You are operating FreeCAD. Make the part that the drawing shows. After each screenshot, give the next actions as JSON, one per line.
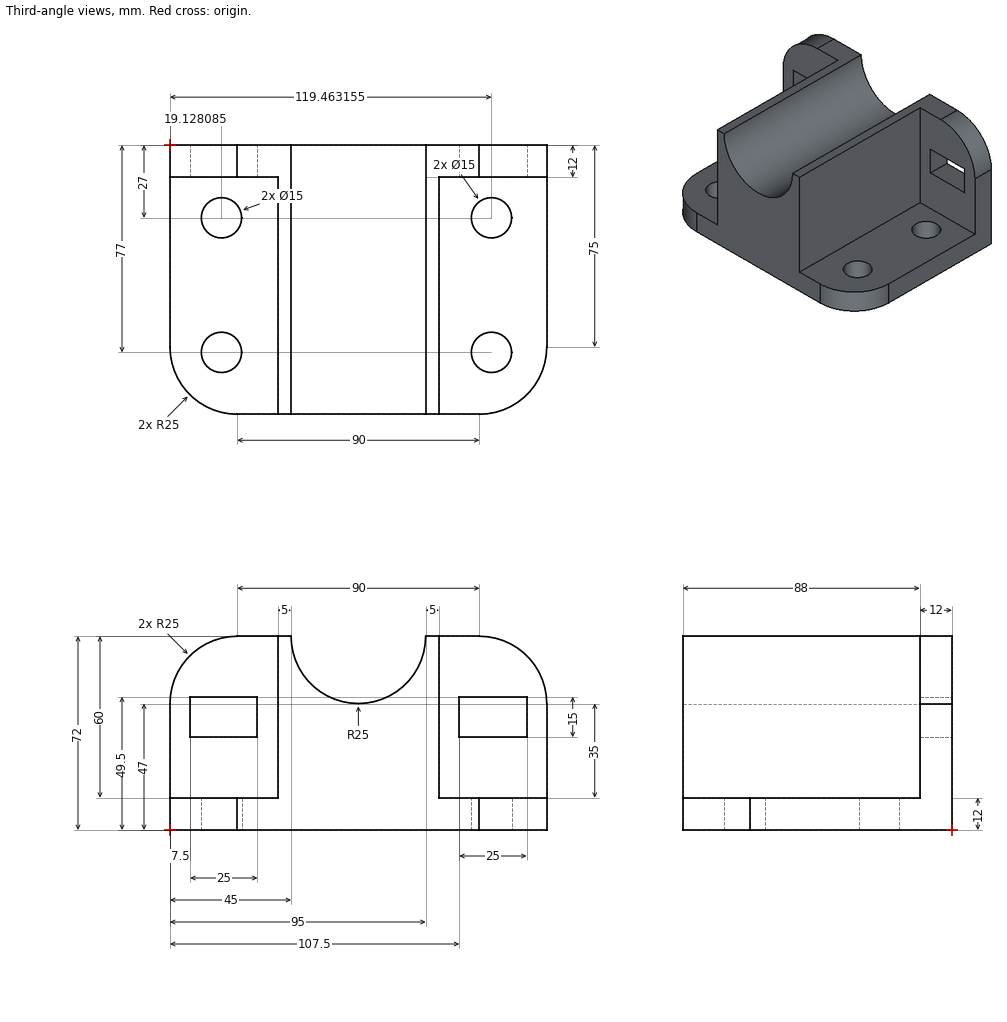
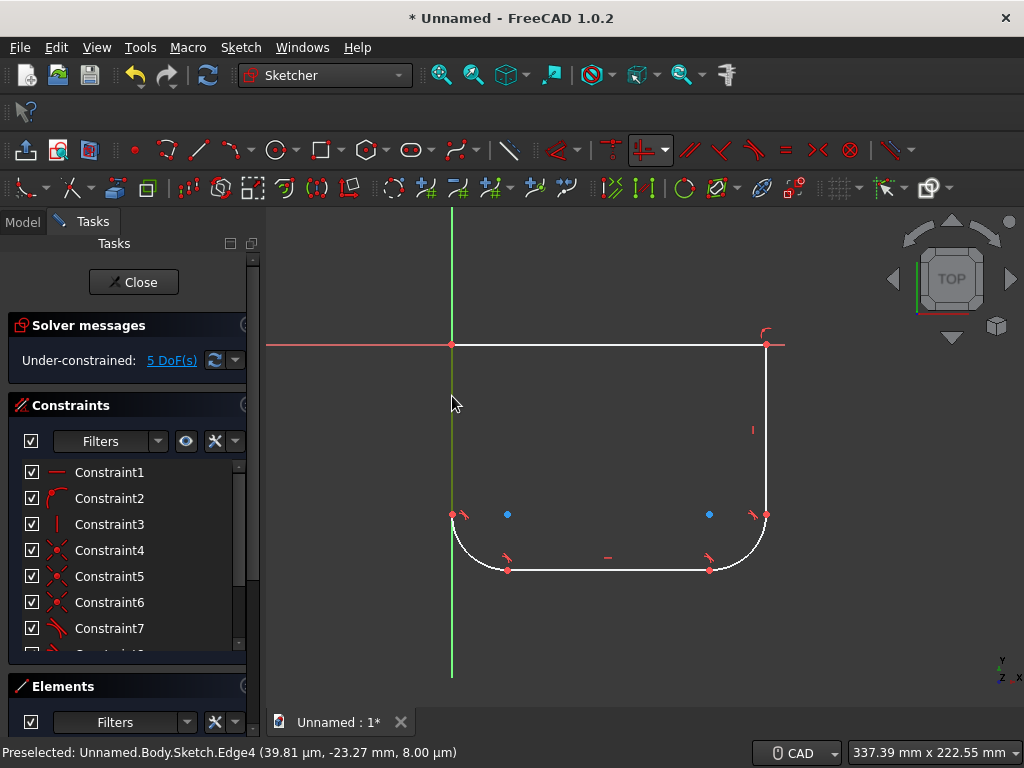
{"action": "key", "text": "v"}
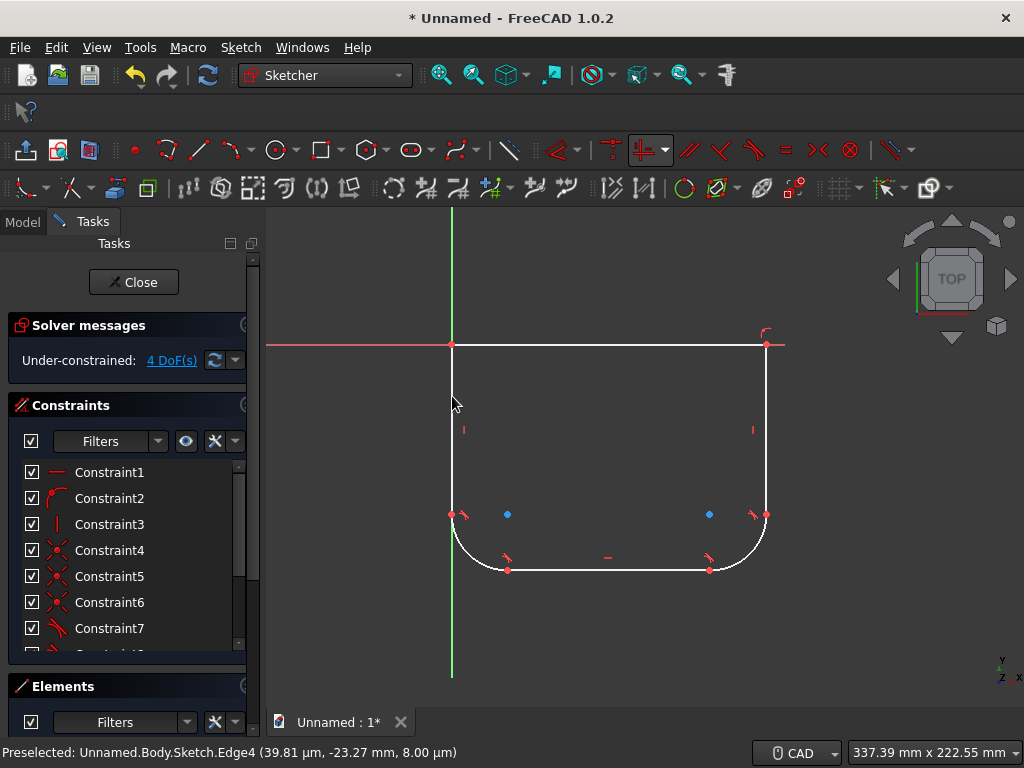
{"action": "left_click", "coordinate": [736, 564]}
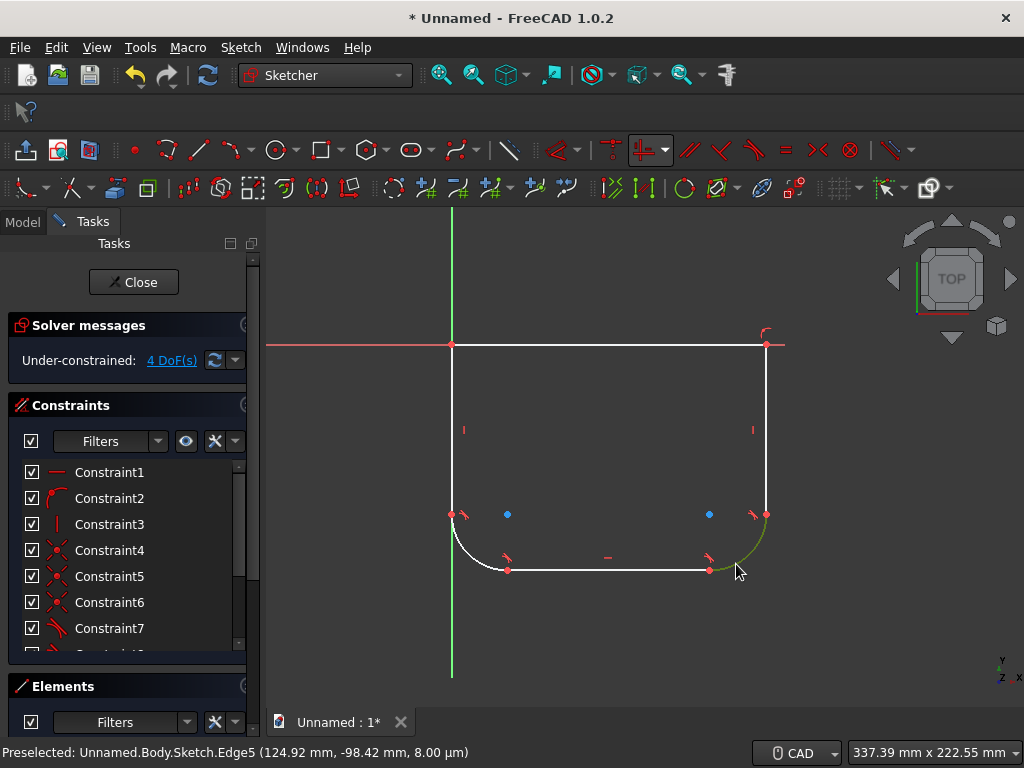
{"action": "left_click", "coordinate": [482, 564]}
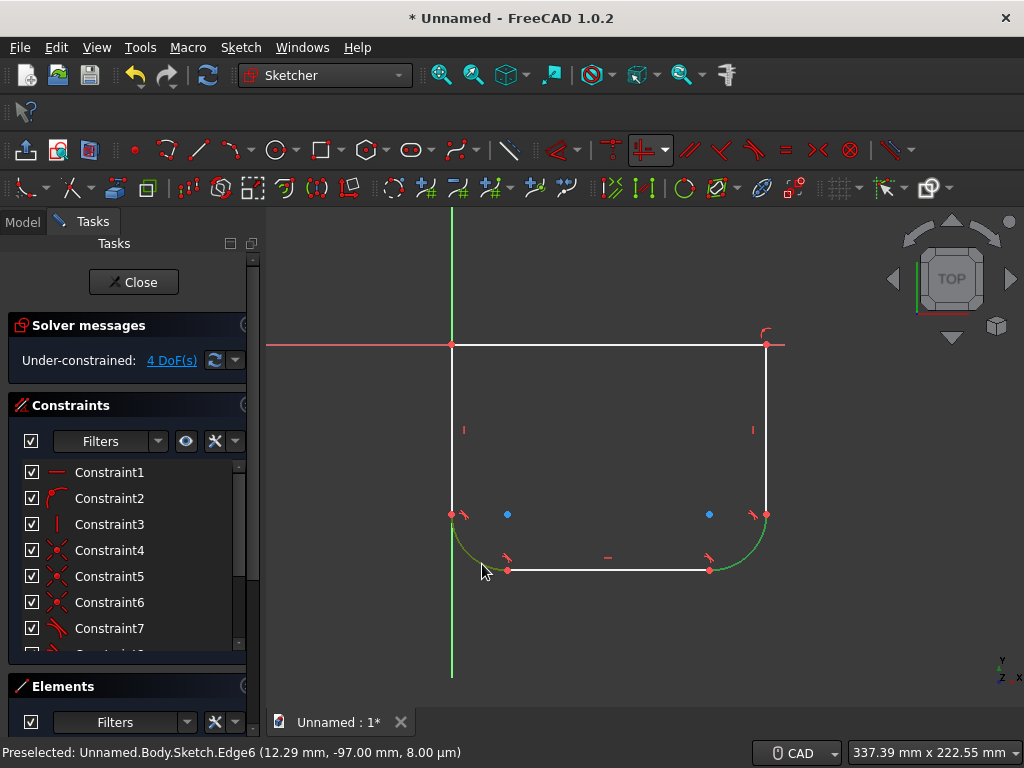
{"action": "key", "text": "e"}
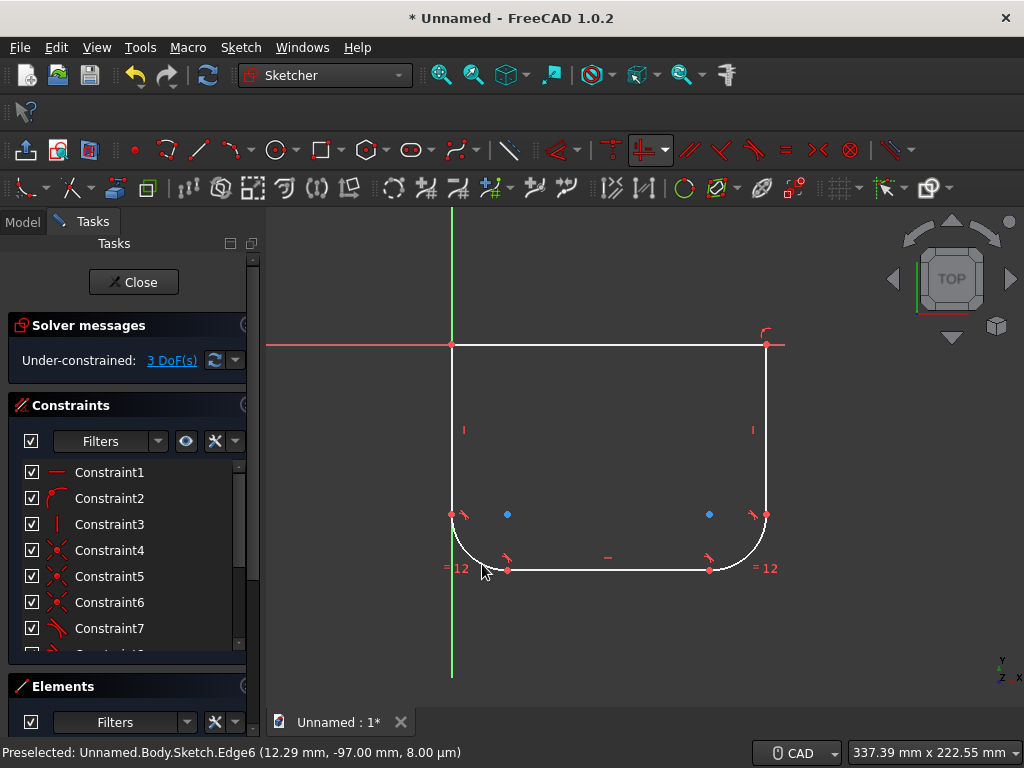
{"action": "left_click", "coordinate": [736, 564]}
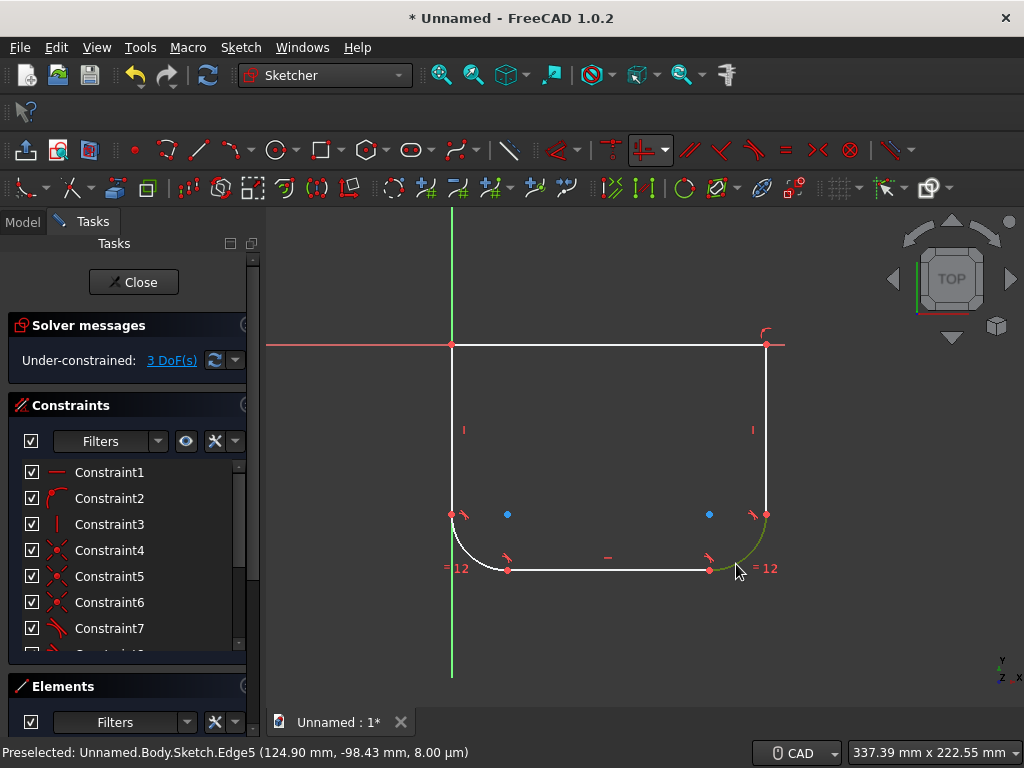
{"action": "key", "text": "k r"}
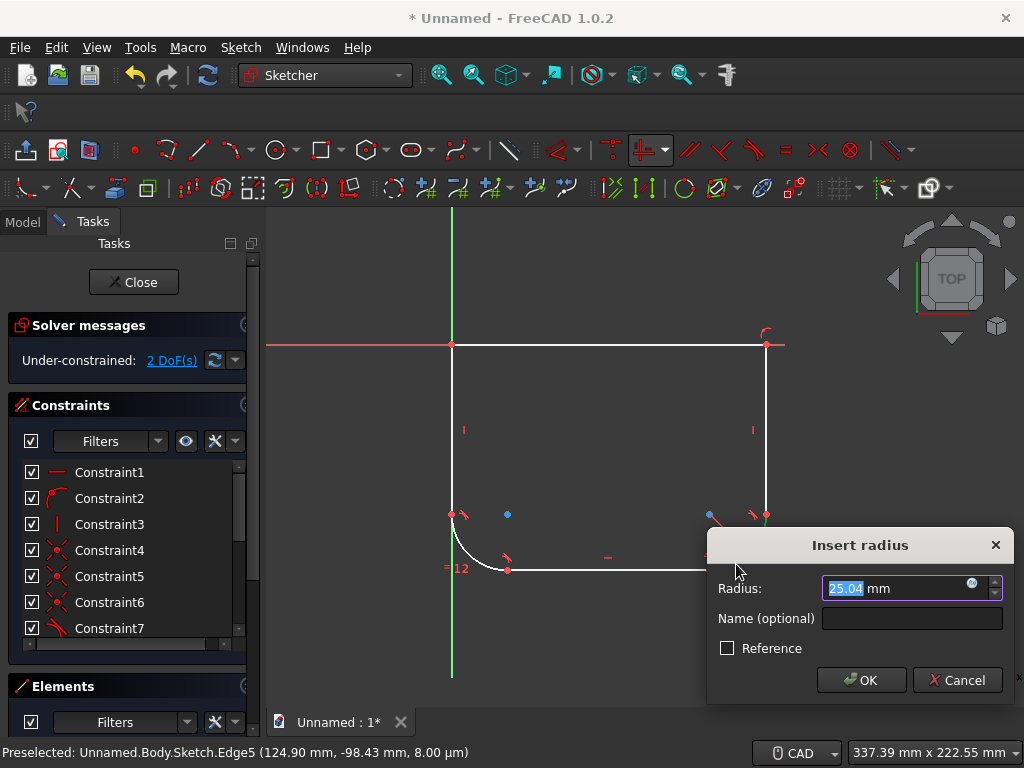
{"action": "type", "text": "25"}
{"action": "key", "text": "Return"}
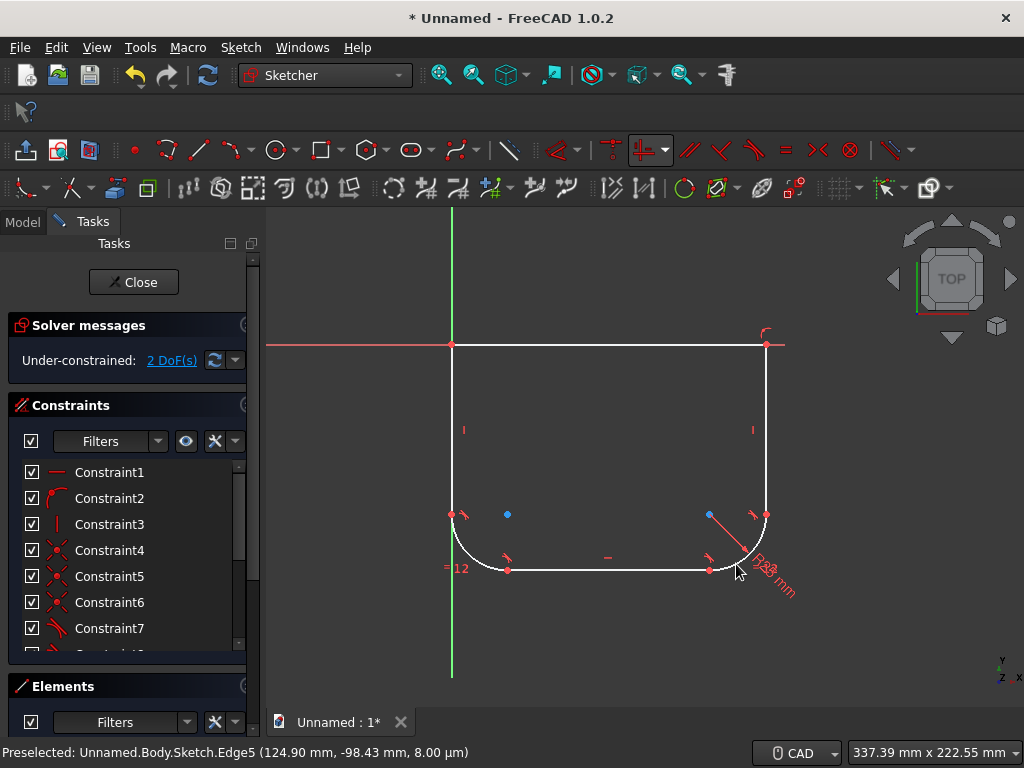
{"action": "left_click", "coordinate": [569, 570]}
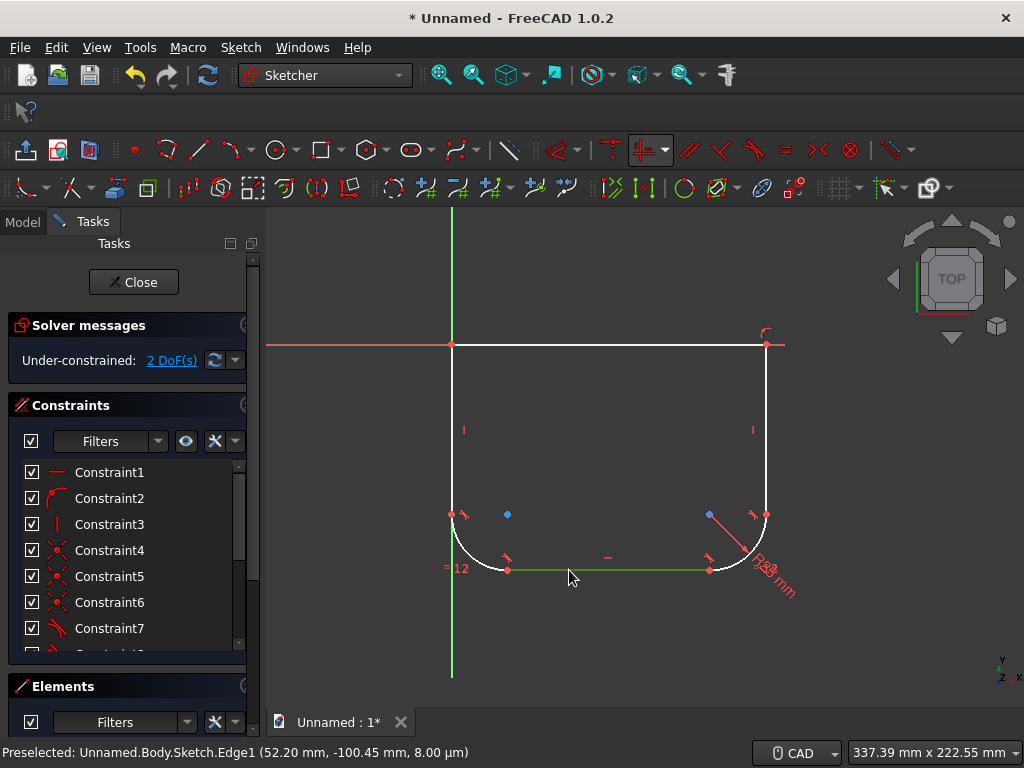
{"action": "key", "text": "l"}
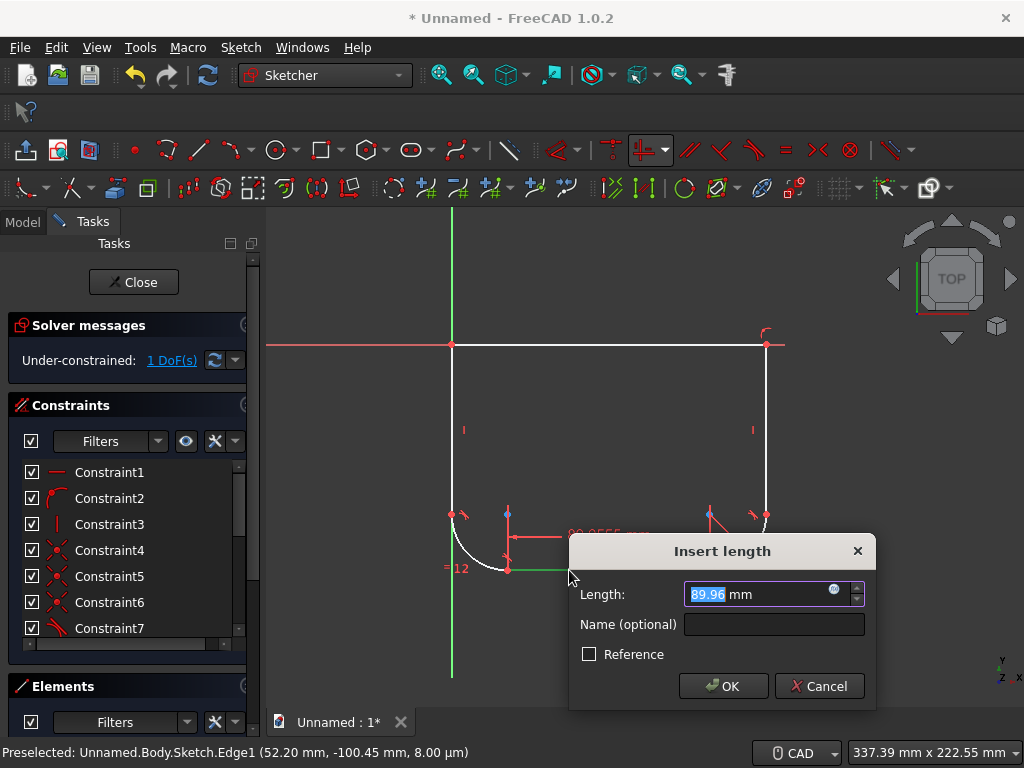
{"action": "type", "text": "90"}
{"action": "key", "text": "Return"}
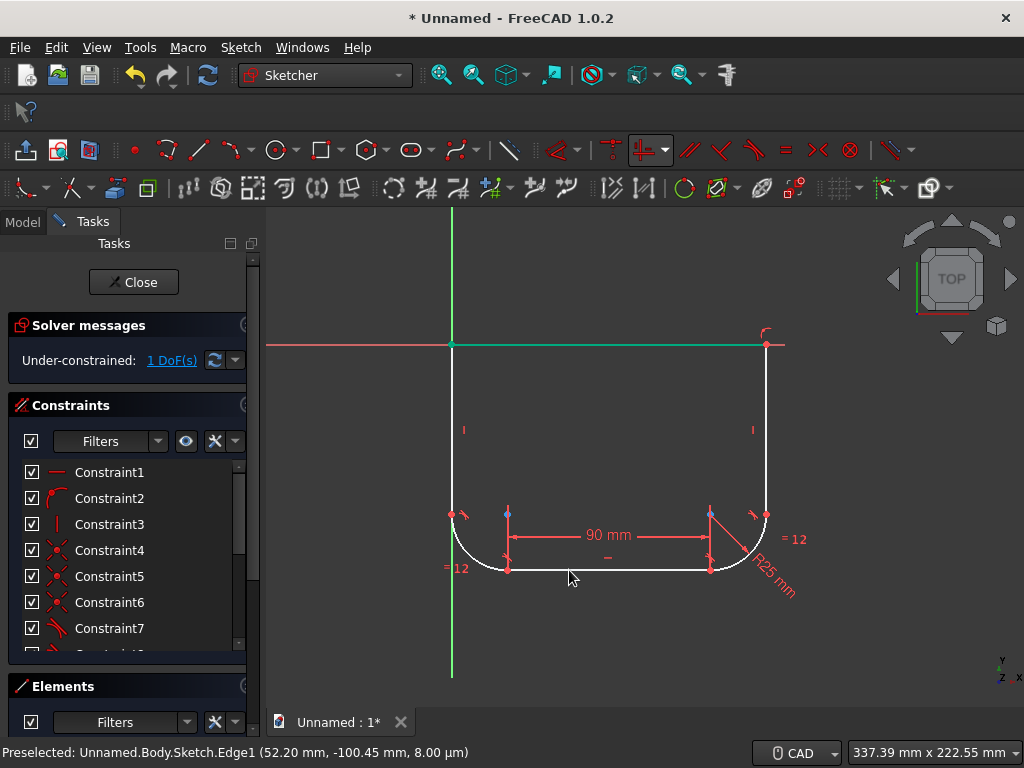
{"action": "left_click", "coordinate": [766, 463]}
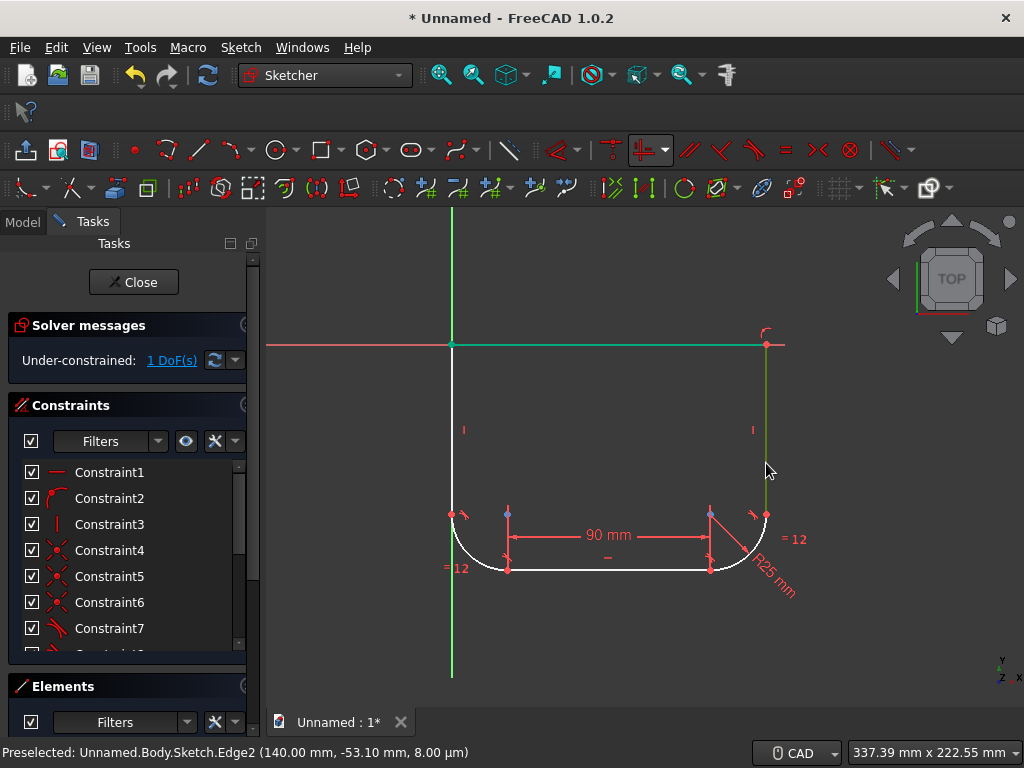
{"action": "key", "text": "i"}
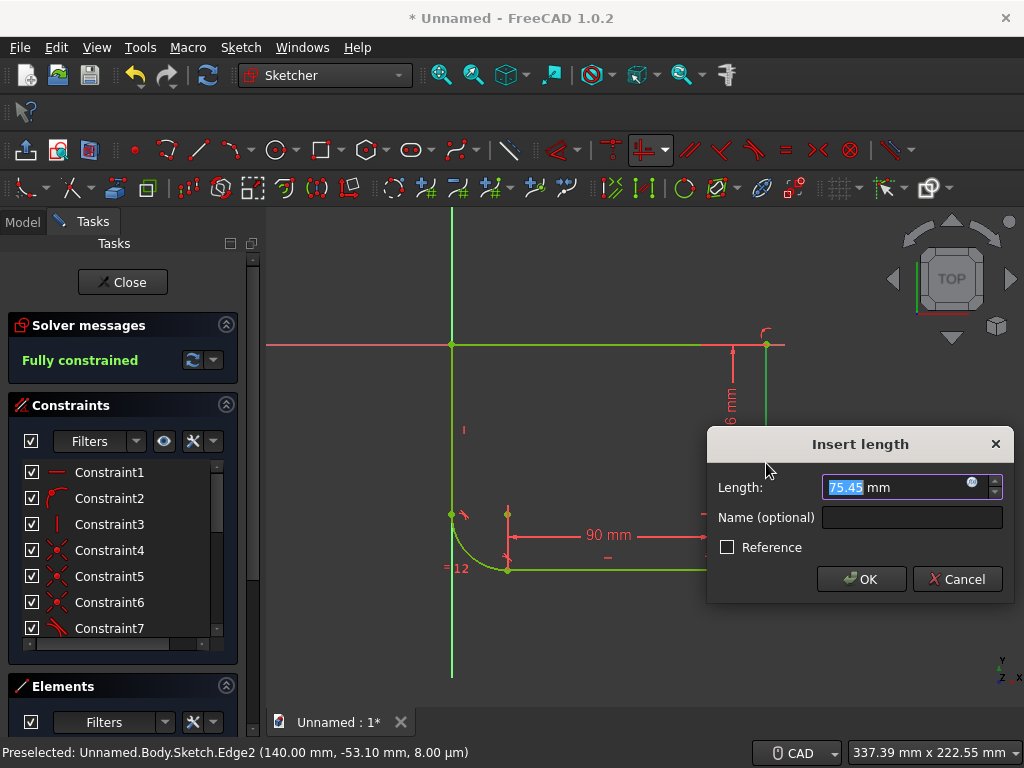
{"action": "type", "text": "75"}
{"action": "key", "text": "Return"}